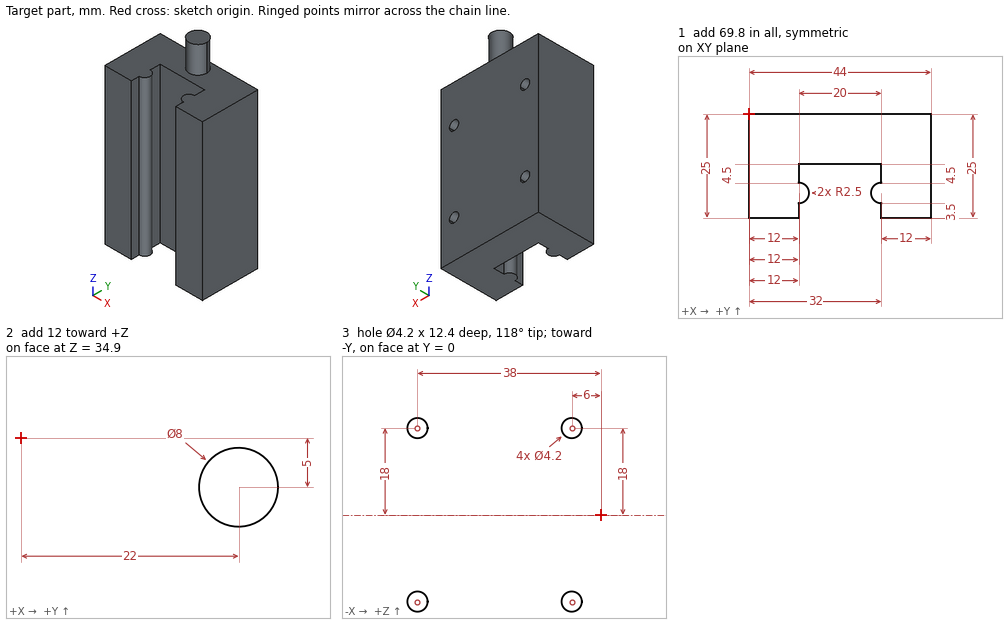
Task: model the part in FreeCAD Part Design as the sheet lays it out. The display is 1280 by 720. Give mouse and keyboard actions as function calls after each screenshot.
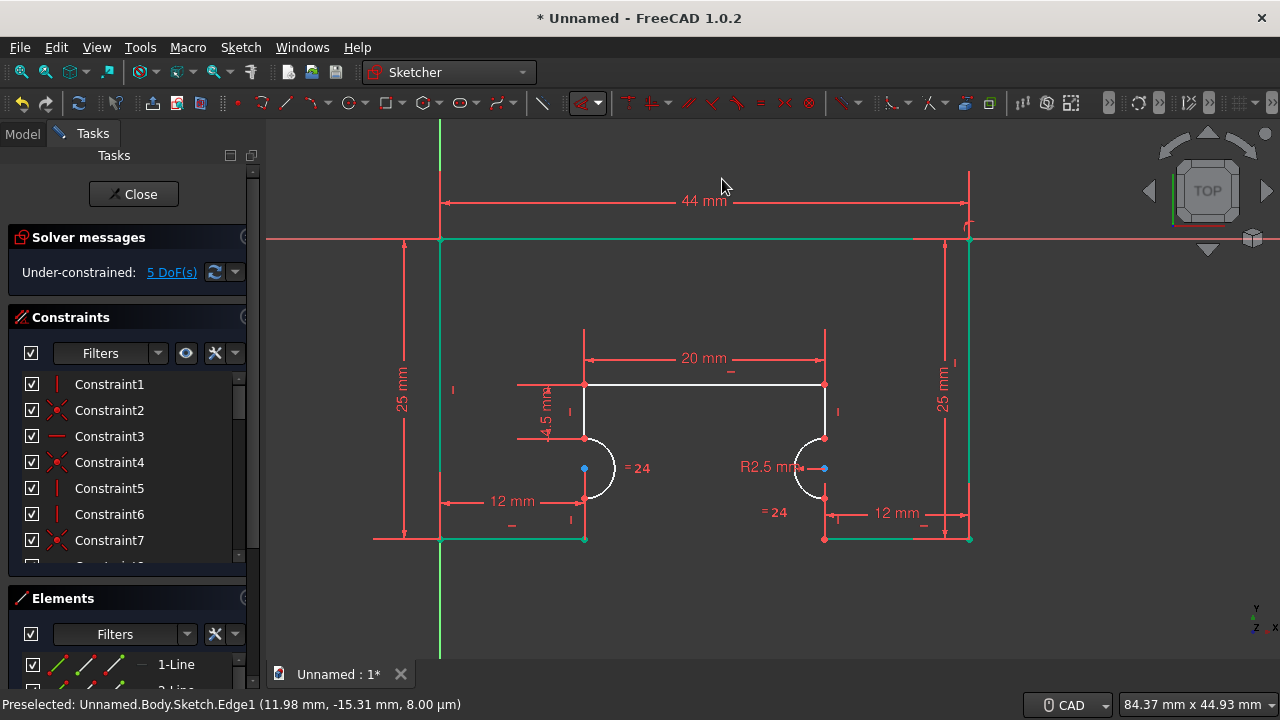
click(825, 401)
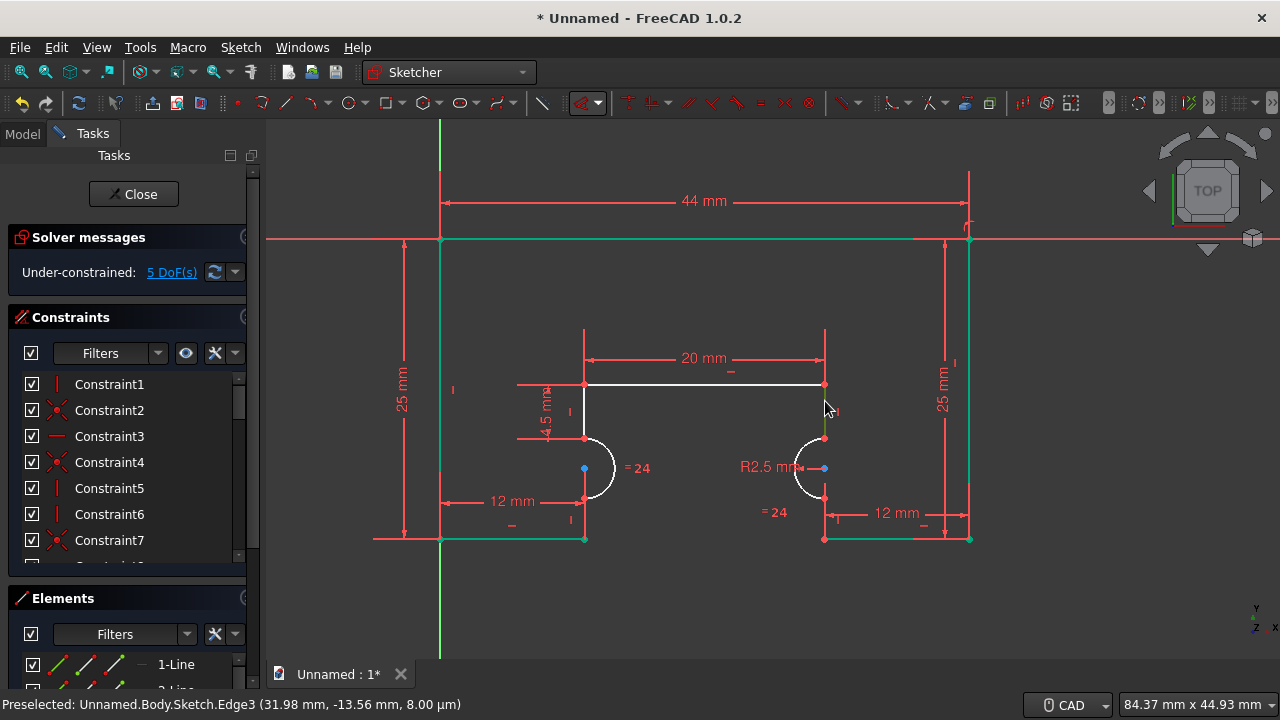
click(600, 104)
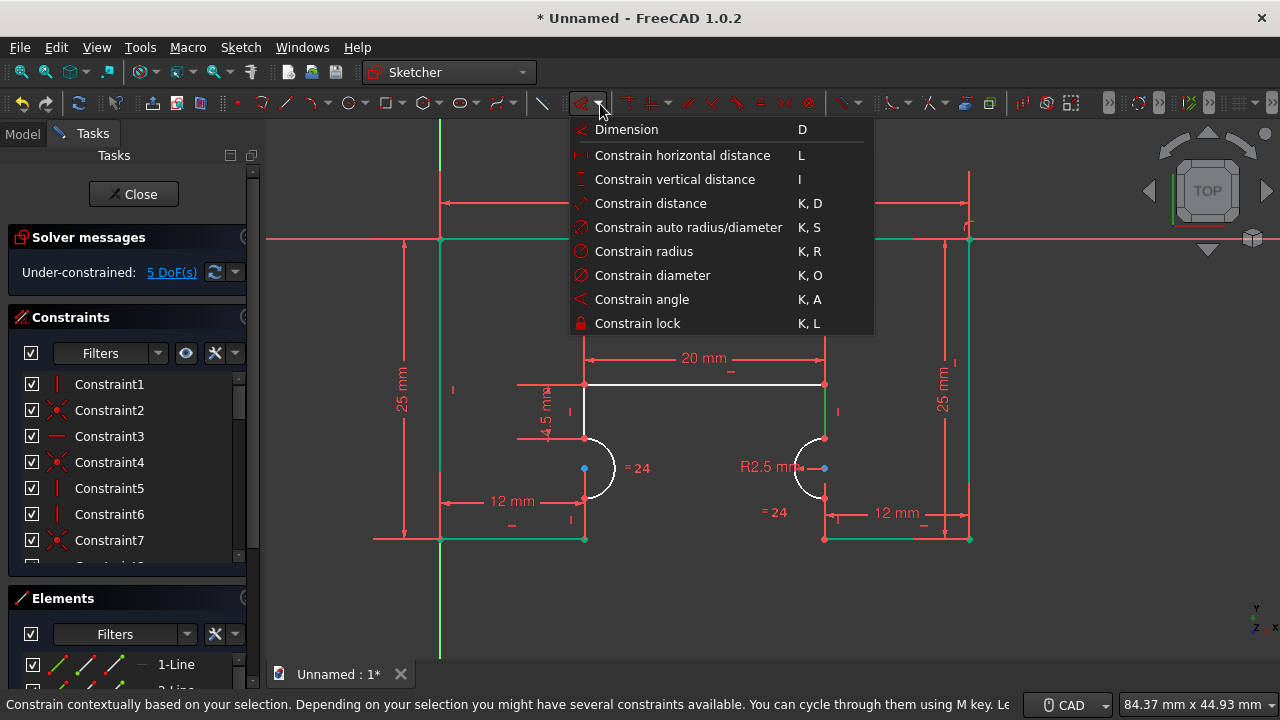
click(722, 179)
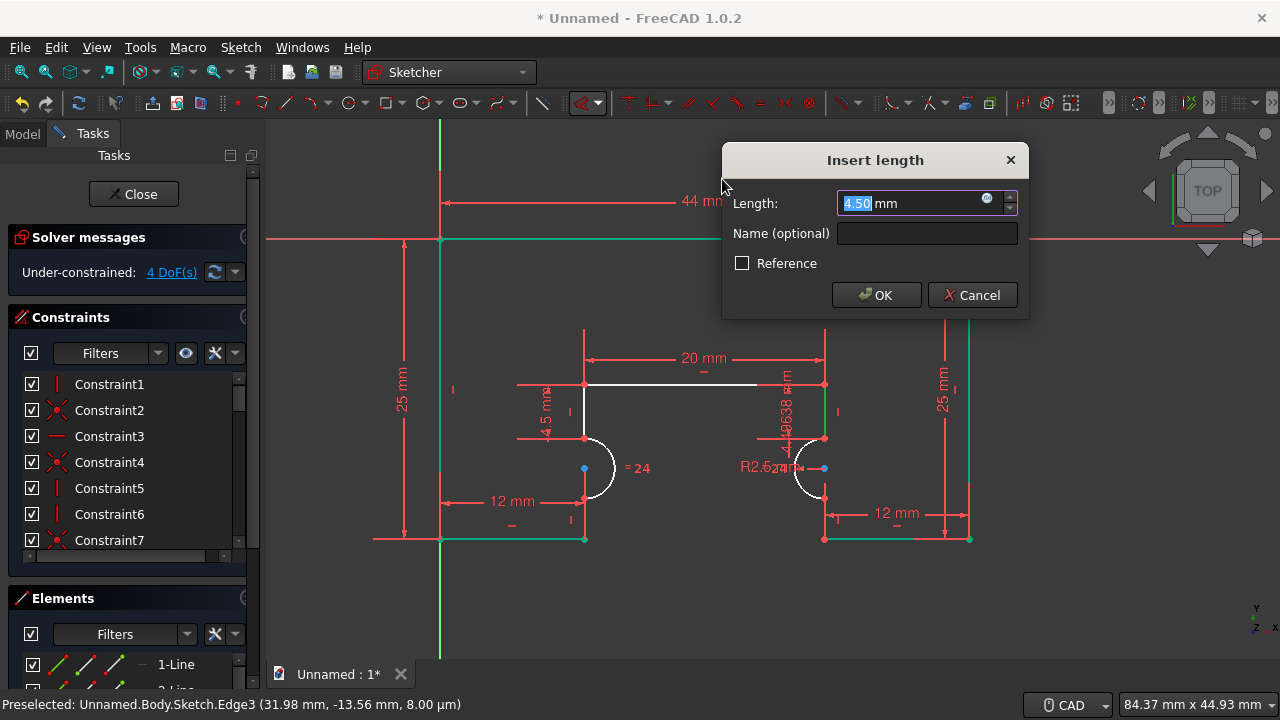
text(4.5)
key(Return)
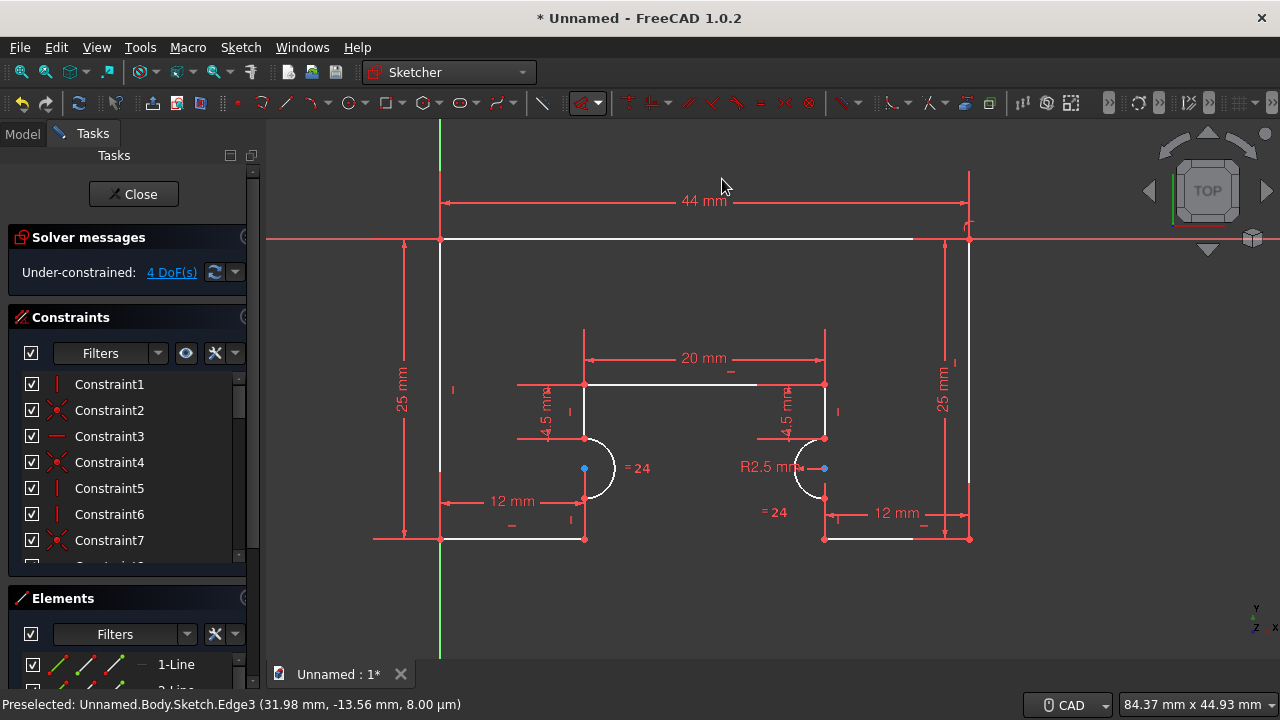
click(825, 511)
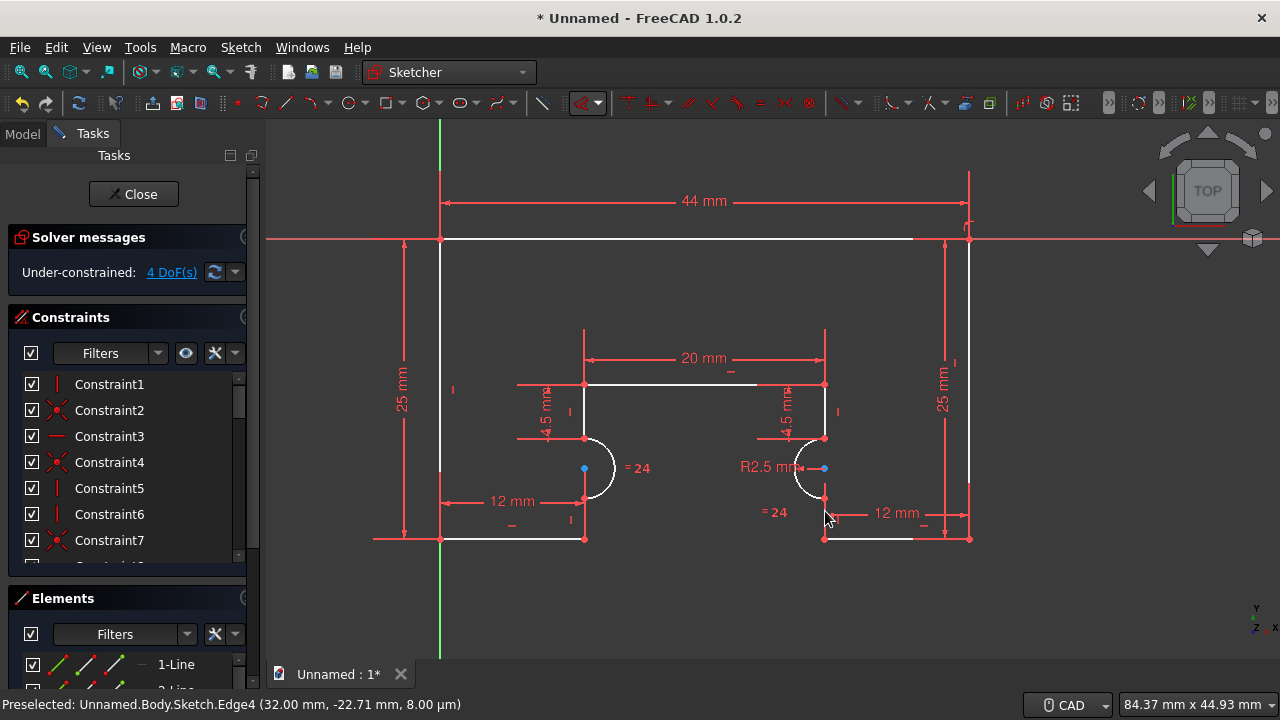
click(600, 104)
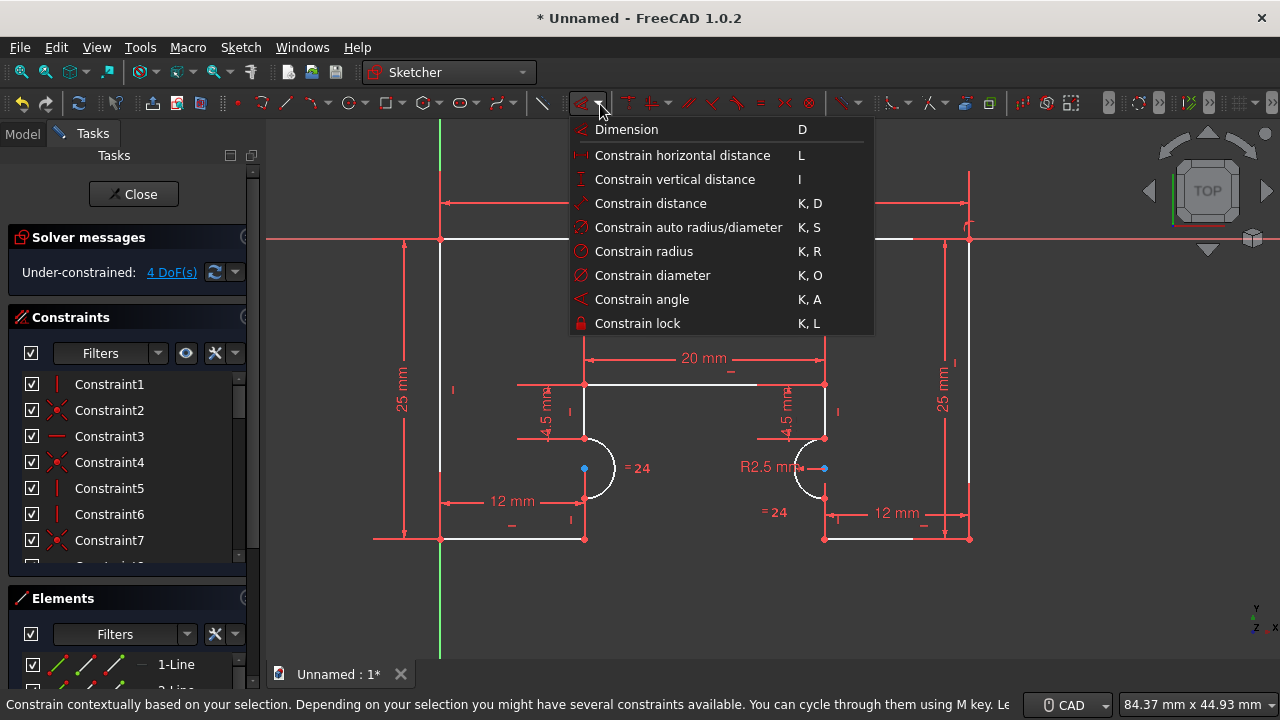
click(722, 179)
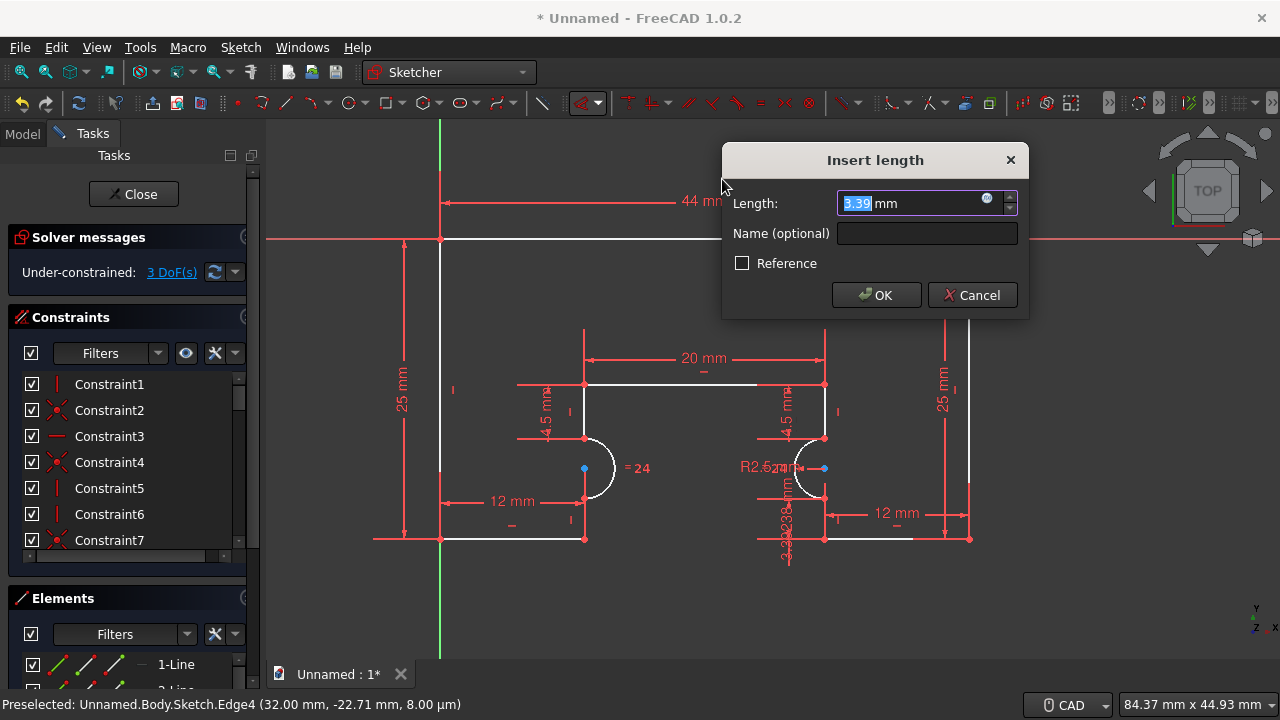
text(3.5)
key(Return)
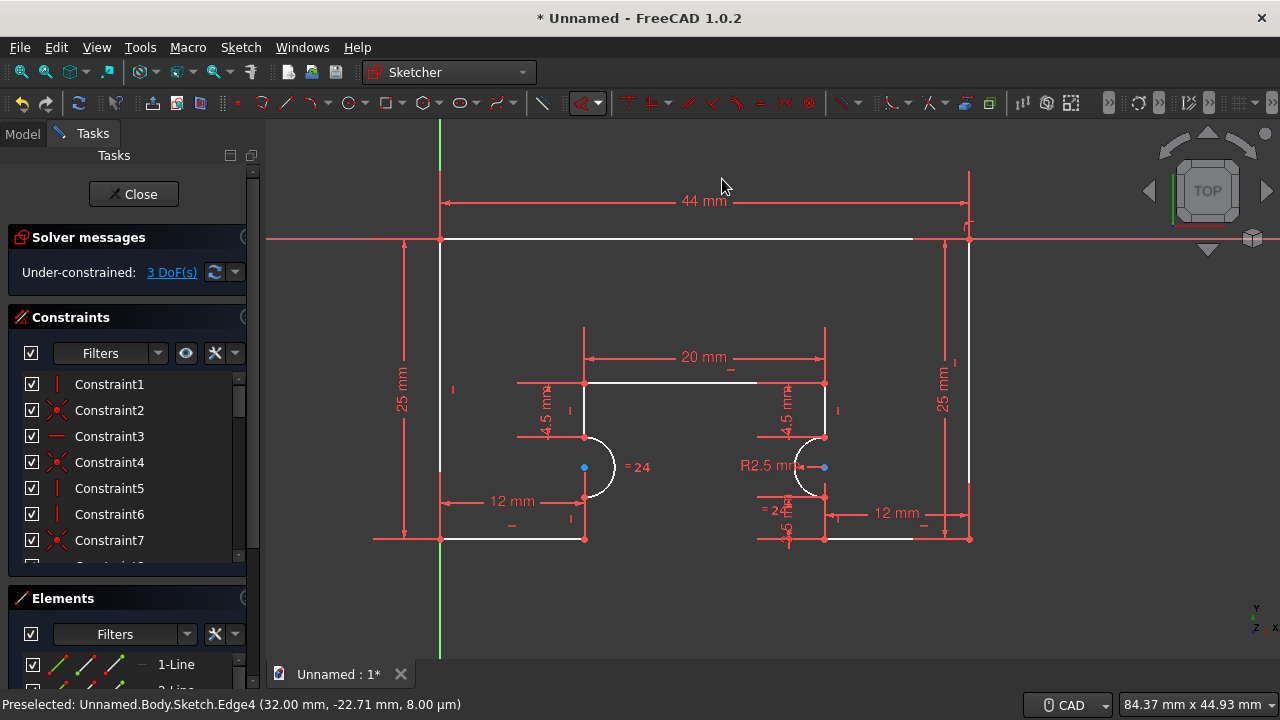
click(584, 437)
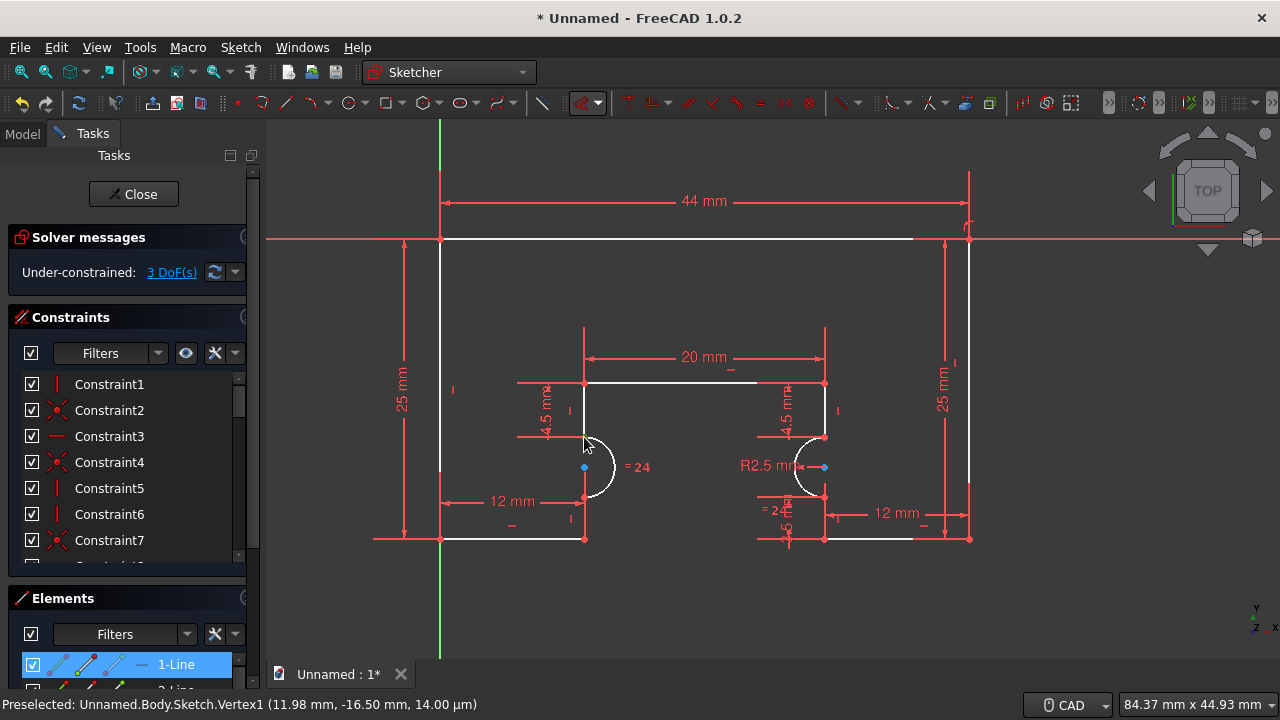
key(l)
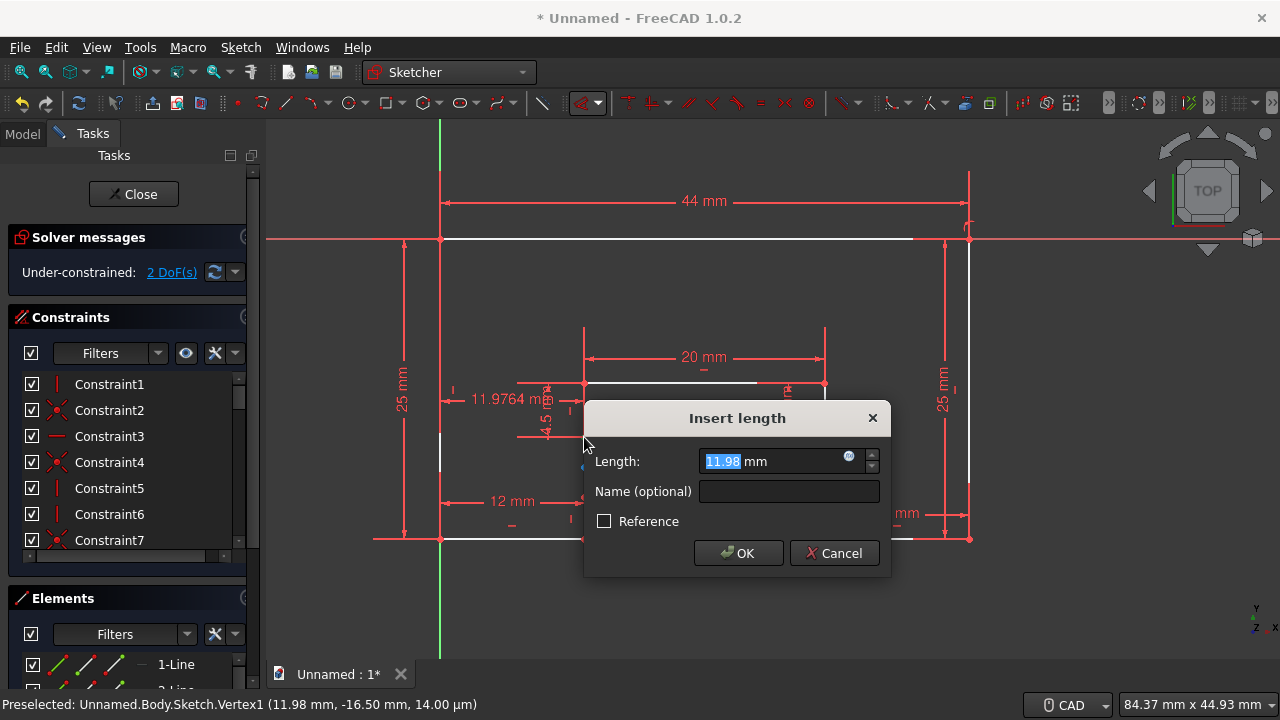
text(12)
key(Return)